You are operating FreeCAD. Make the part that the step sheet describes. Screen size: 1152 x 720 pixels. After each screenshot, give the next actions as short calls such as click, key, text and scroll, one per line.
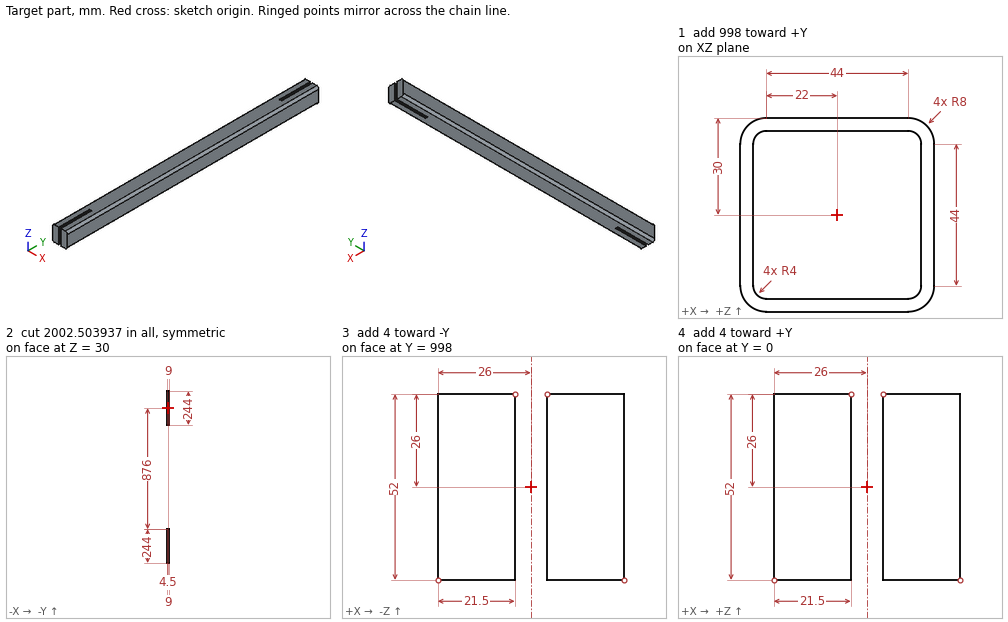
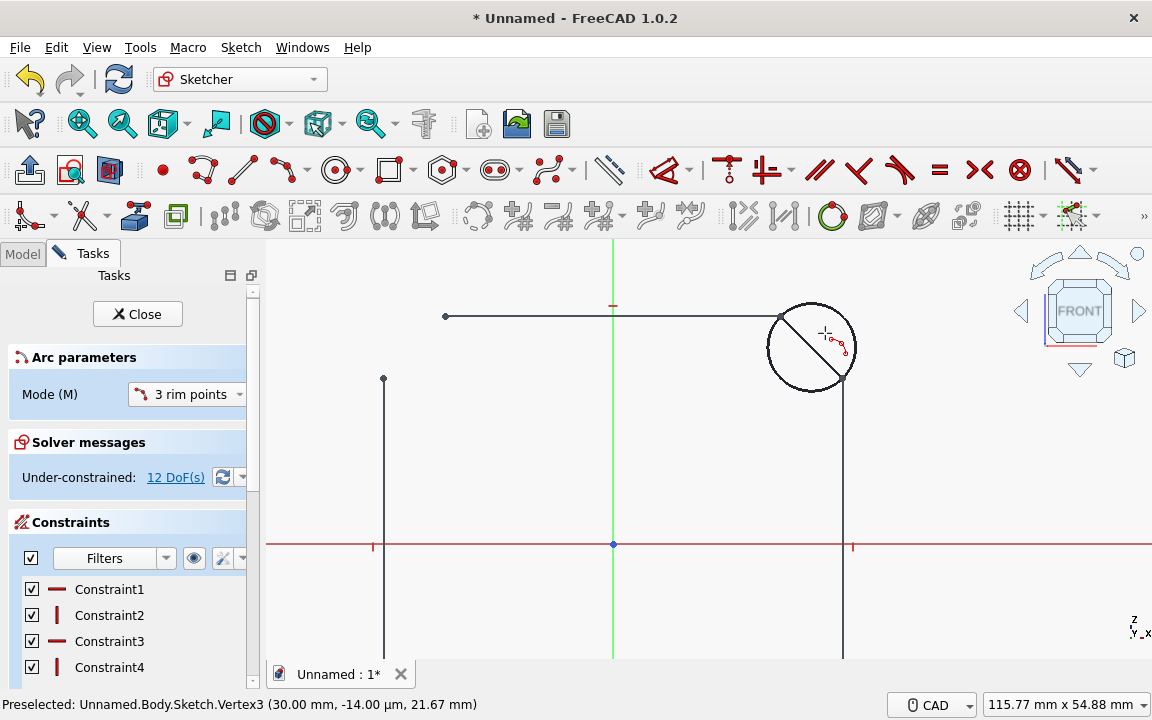
click(825, 333)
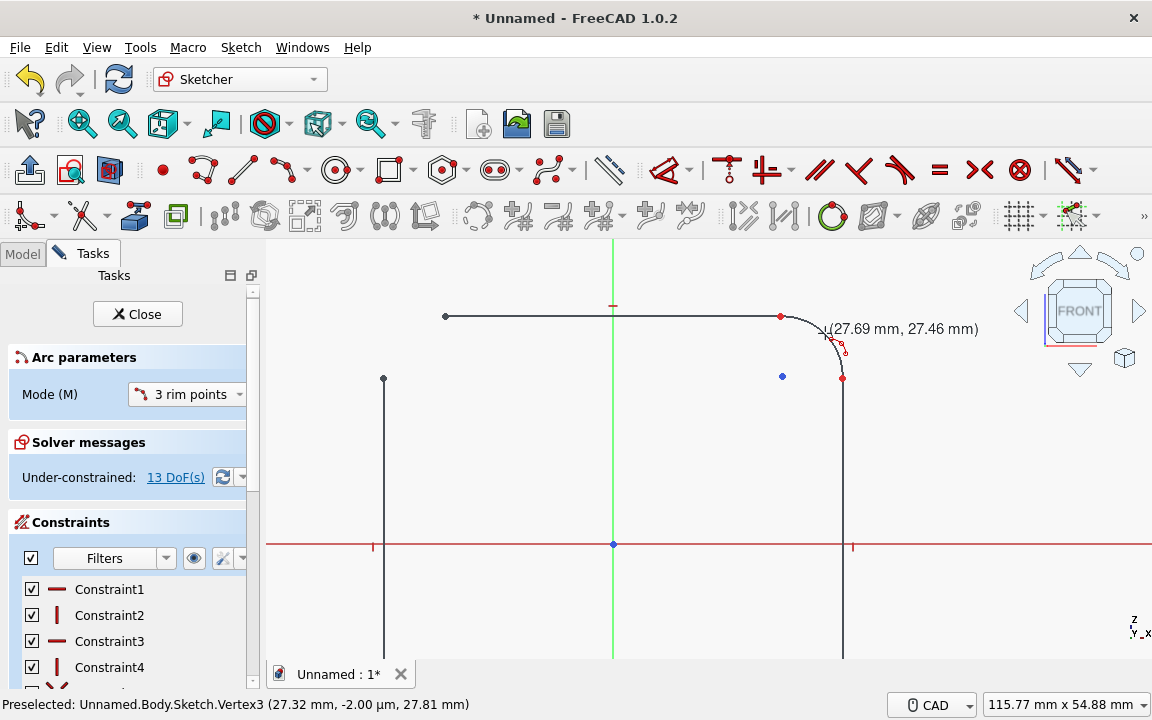
scroll(674, 333, down, 3)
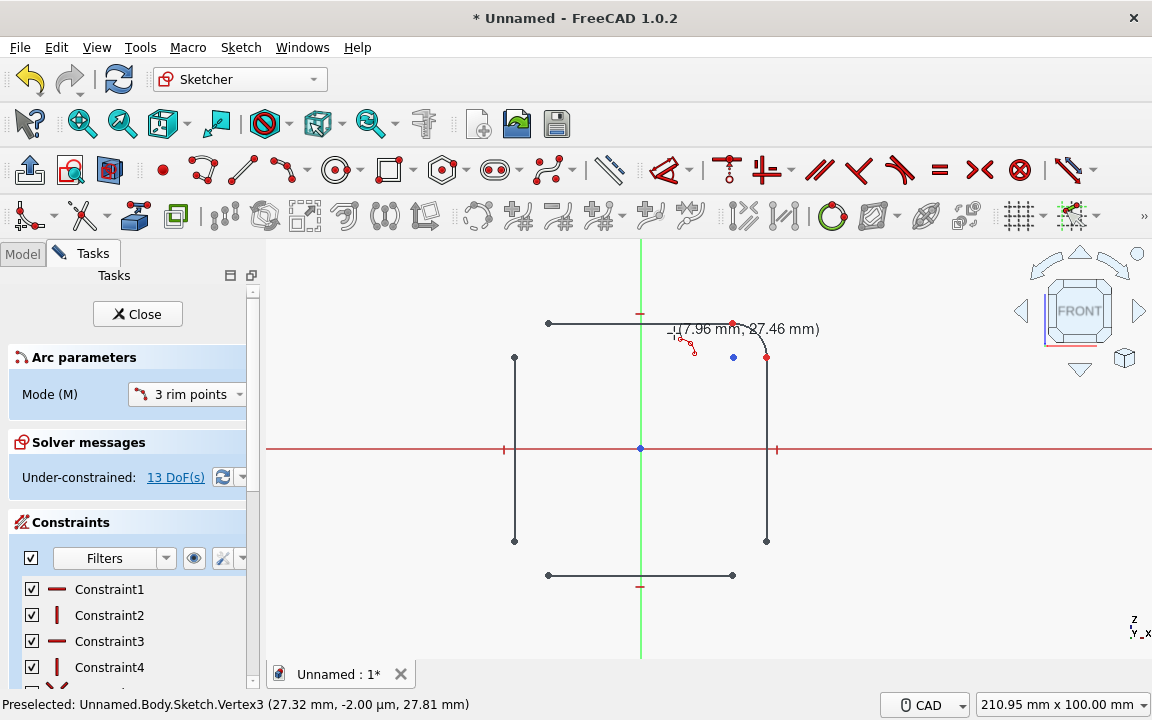
click(767, 542)
click(733, 576)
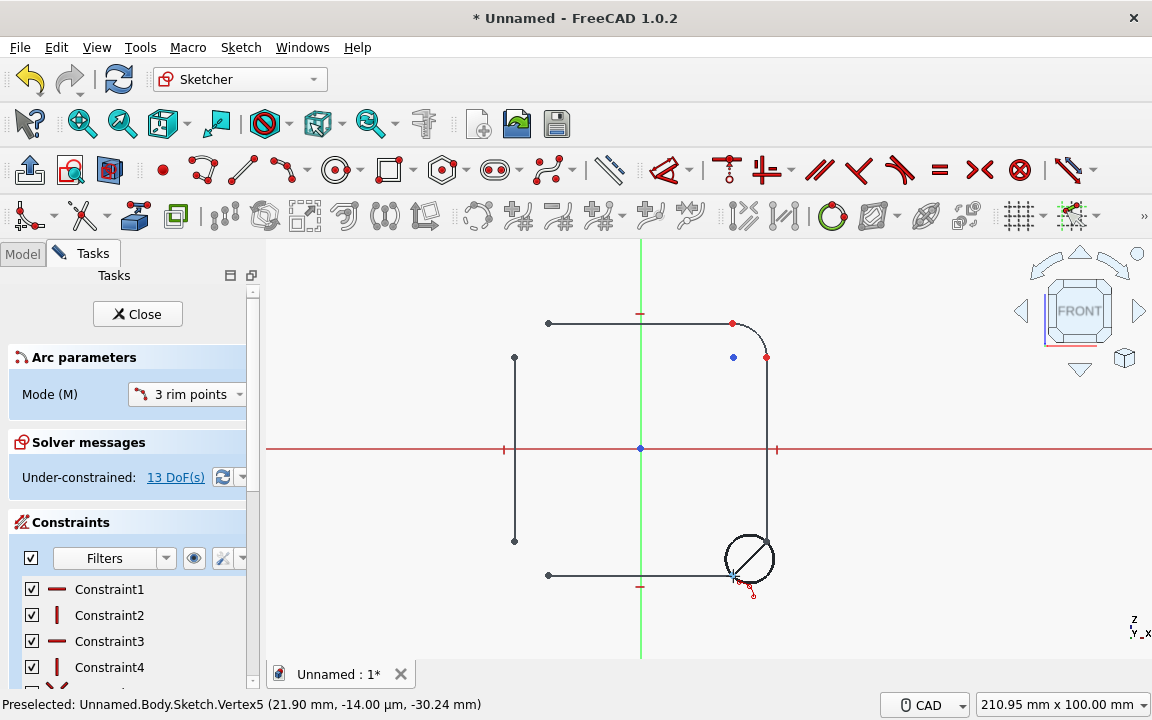
scroll(757, 565, up, 3)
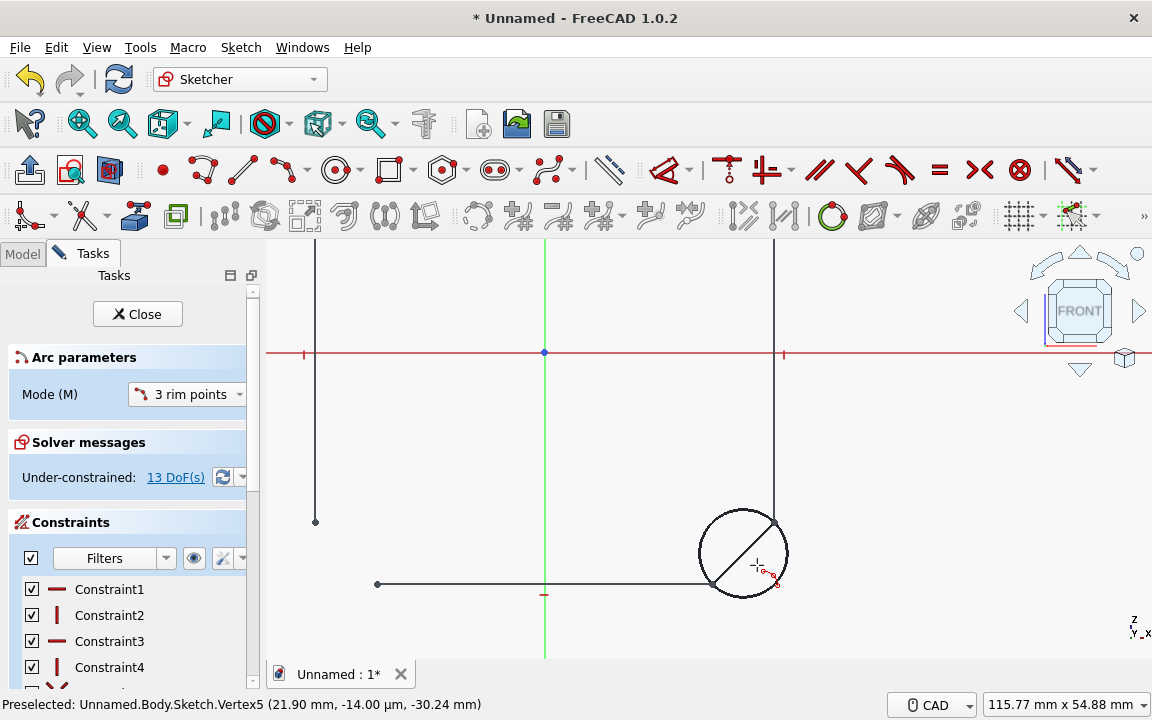
click(756, 565)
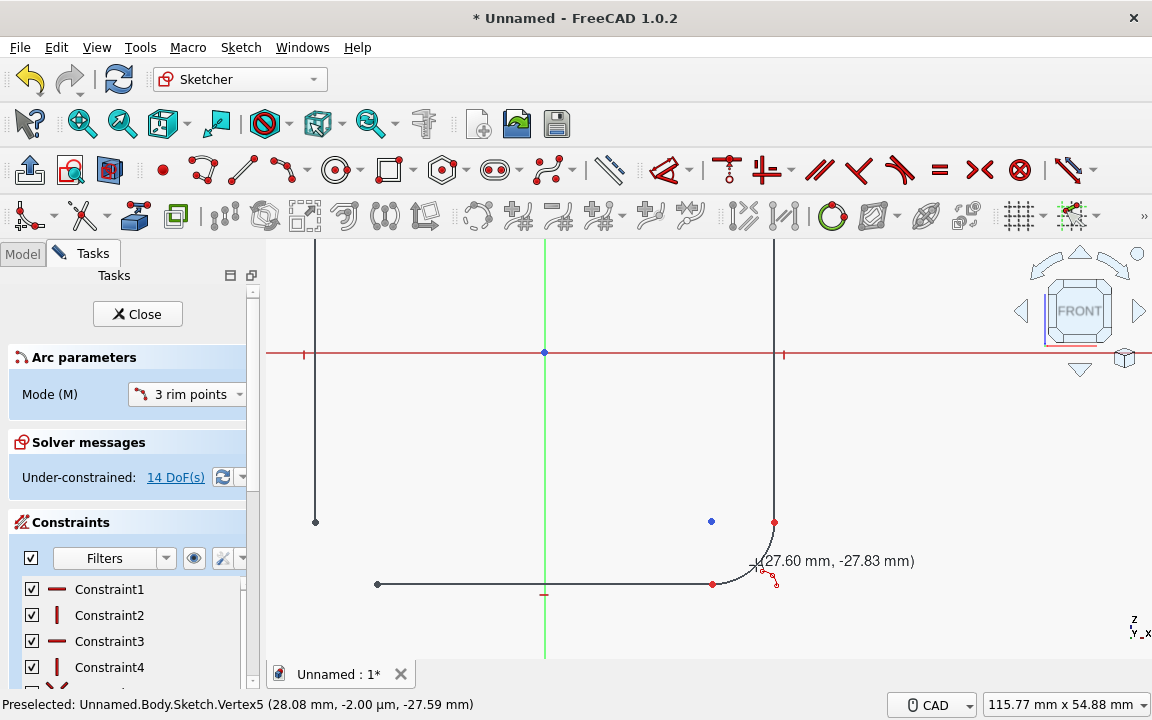
click(377, 584)
click(315, 522)
click(333, 565)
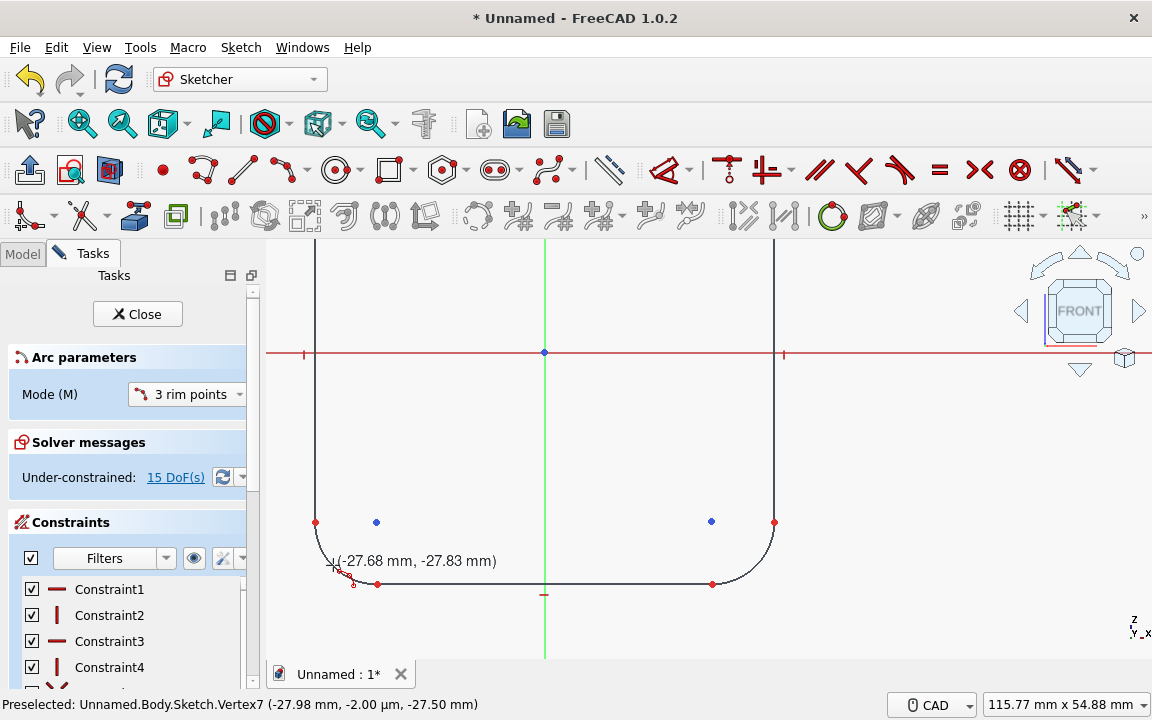
scroll(757, 566, down, 3)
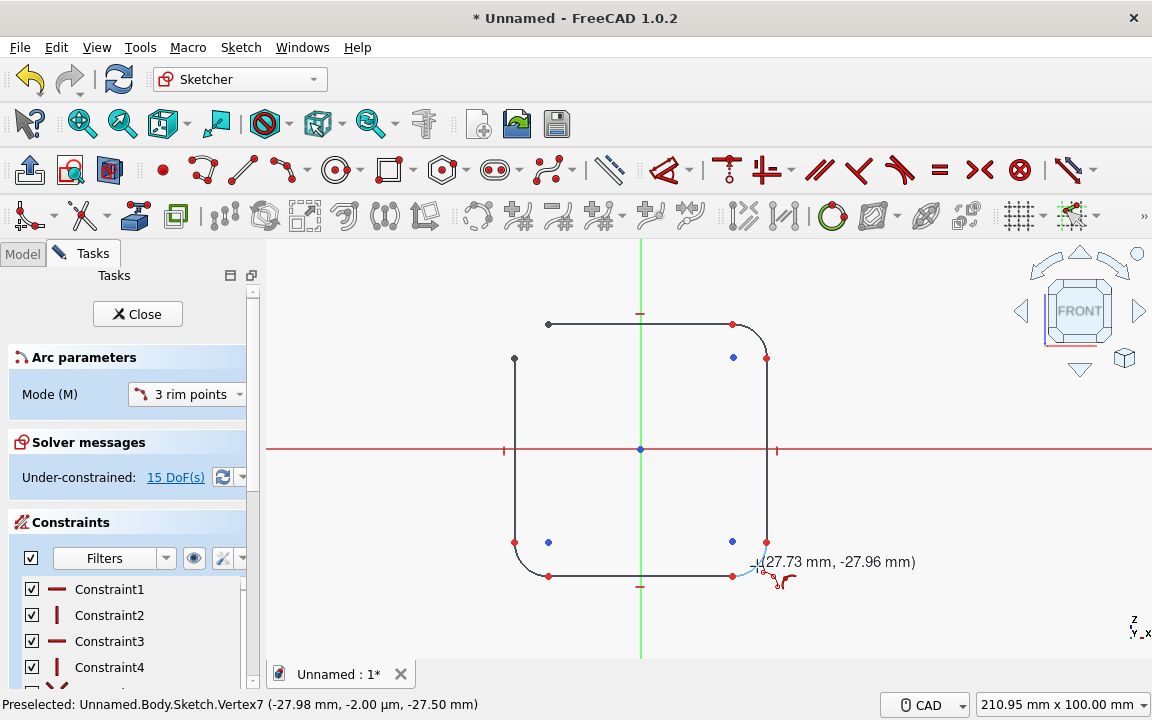
click(515, 358)
click(549, 324)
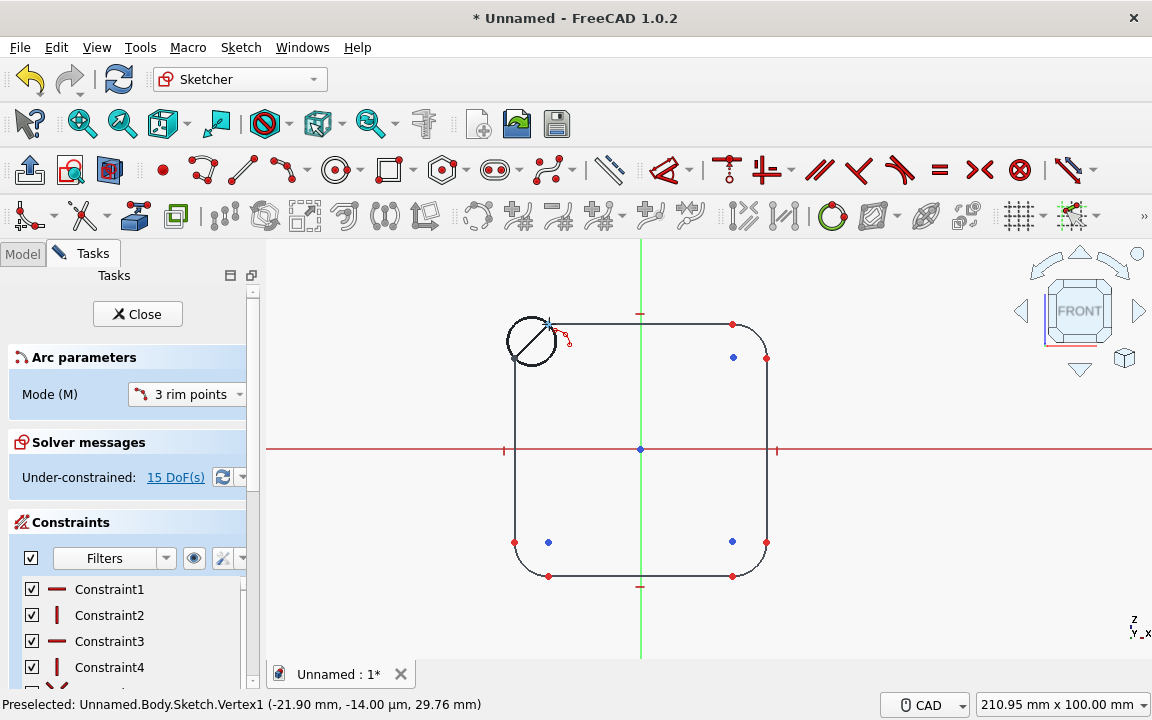
scroll(525, 333, up, 3)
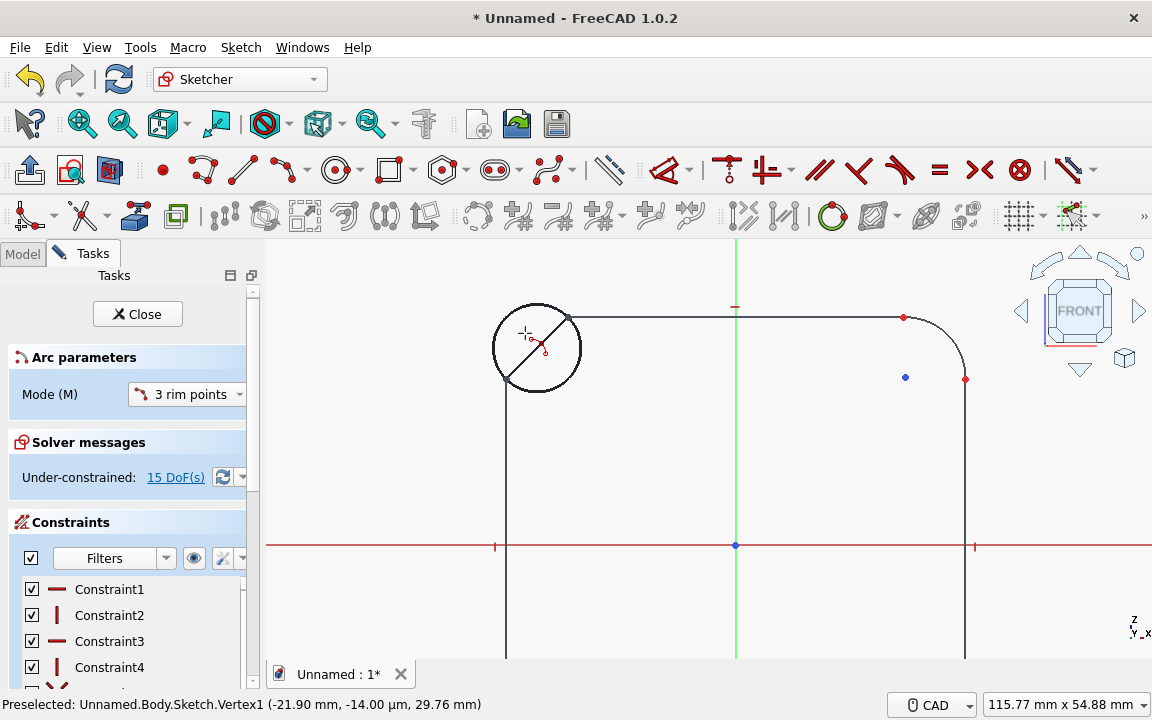
click(524, 333)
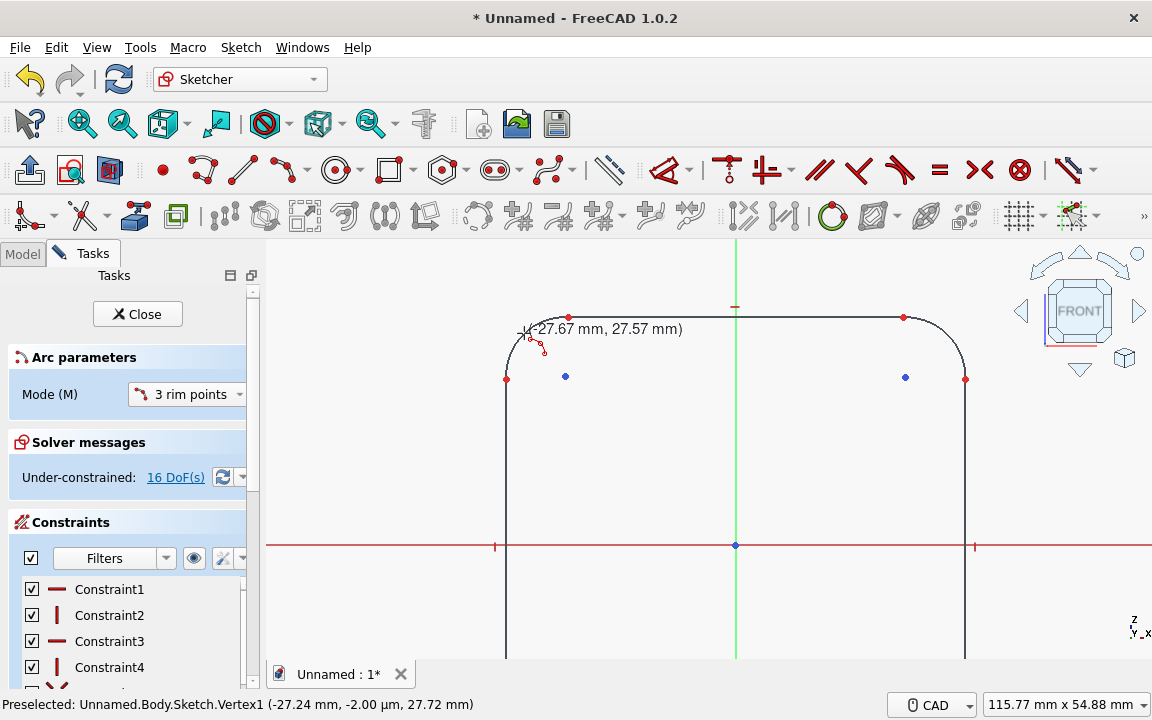
click(244, 170)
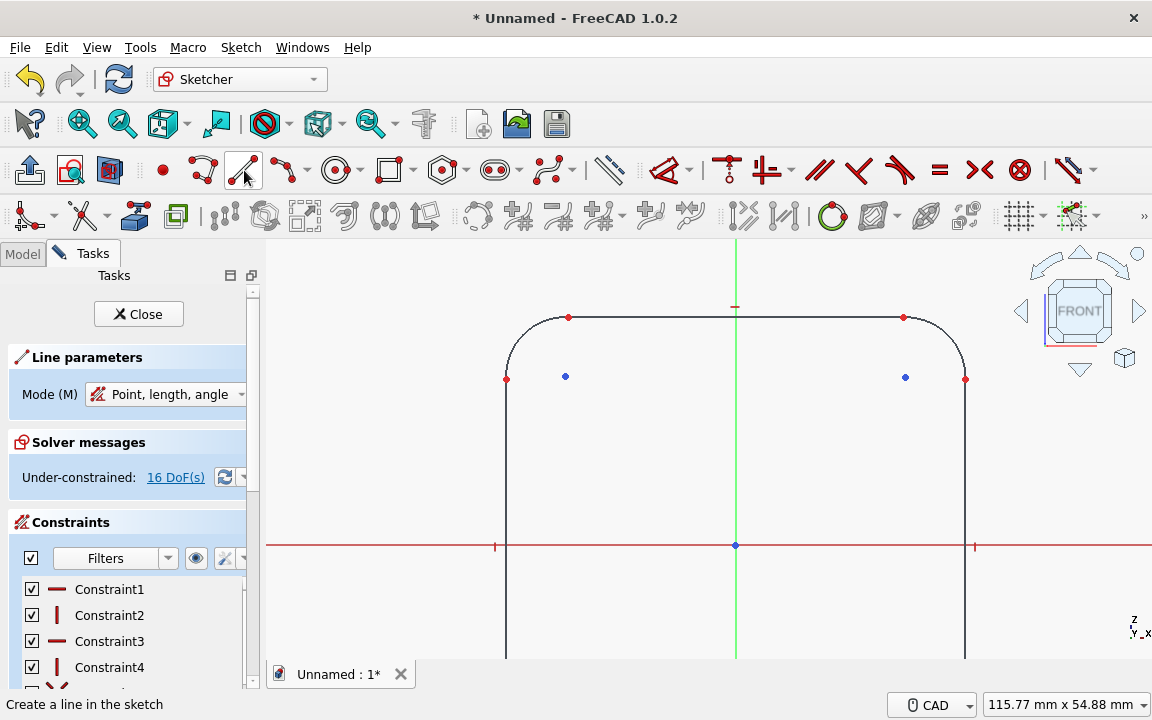
scroll(525, 332, down, 3)